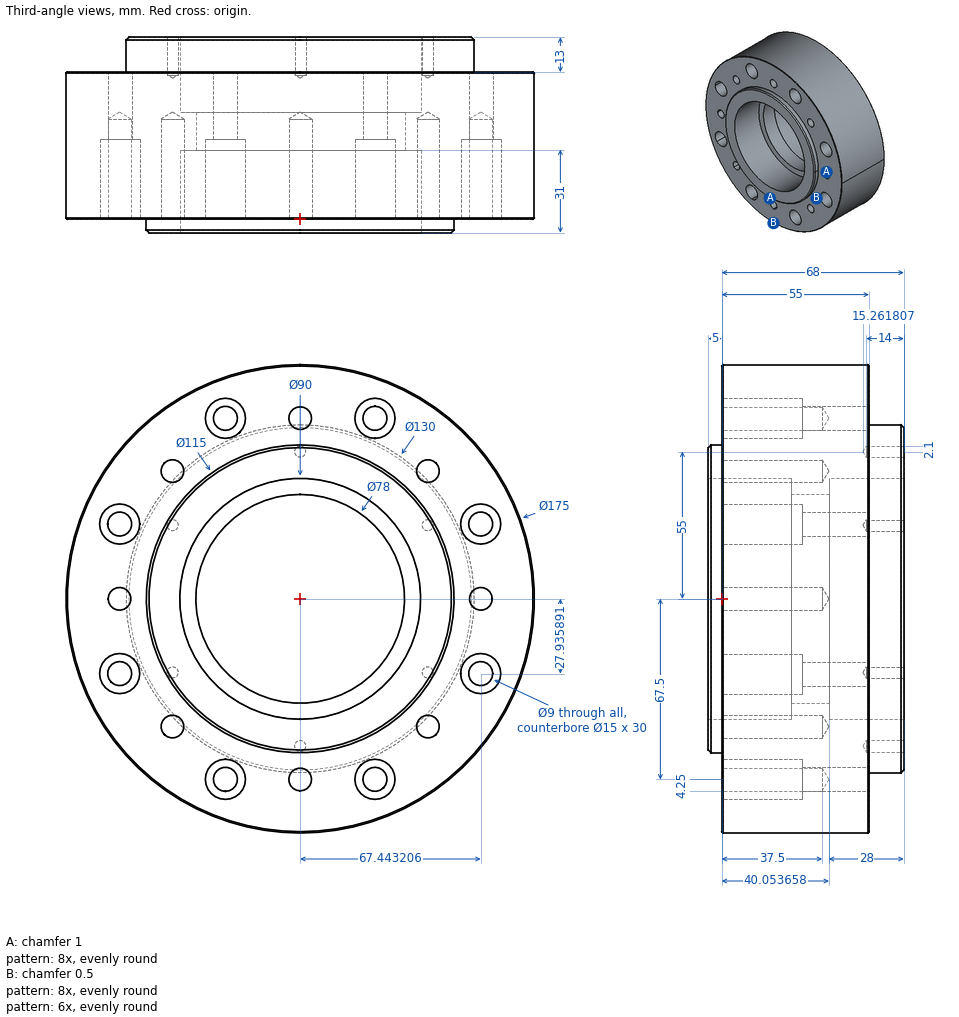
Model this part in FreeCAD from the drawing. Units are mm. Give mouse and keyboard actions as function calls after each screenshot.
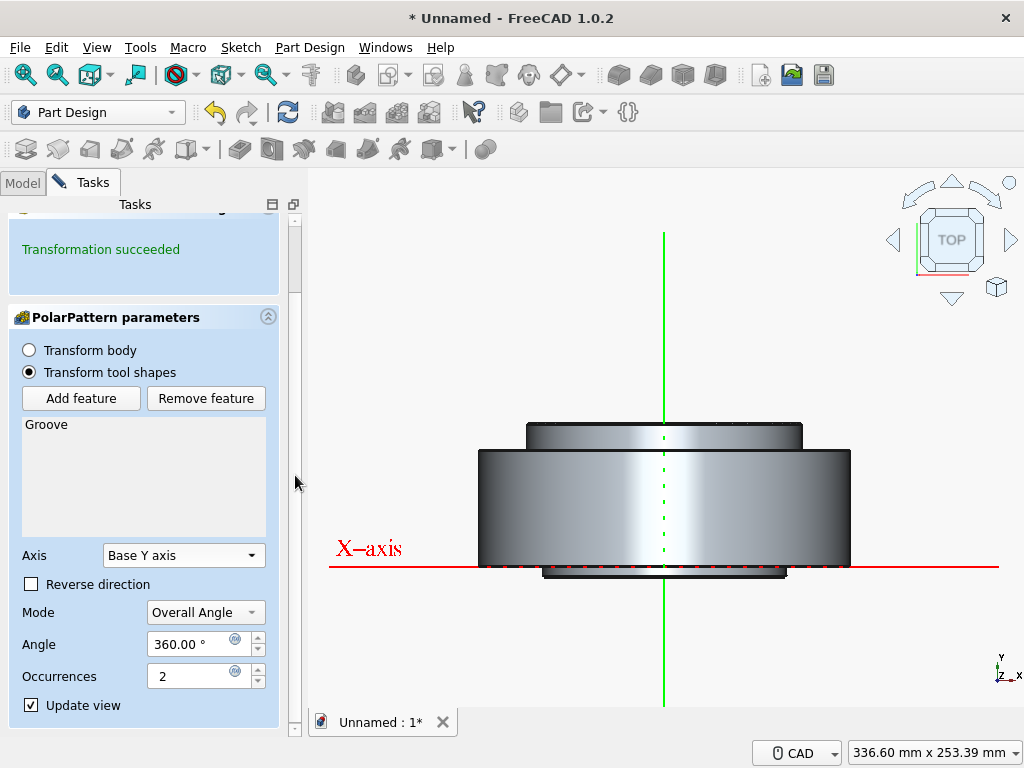
triple_click(198, 676)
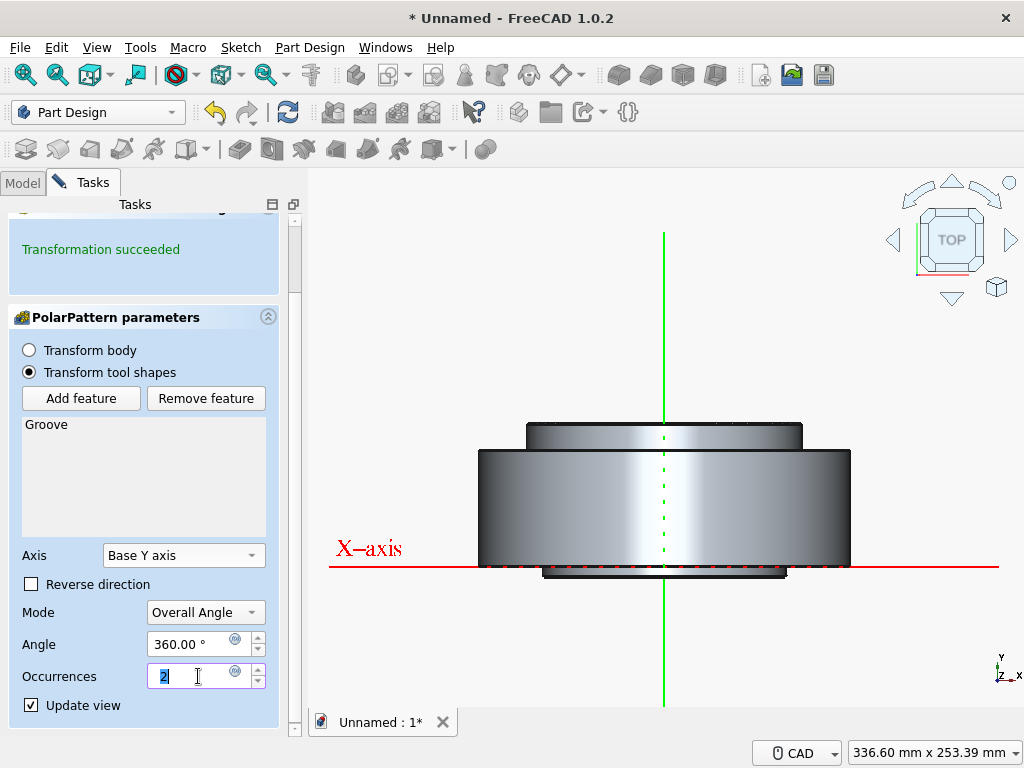
text(8)
key(Tab)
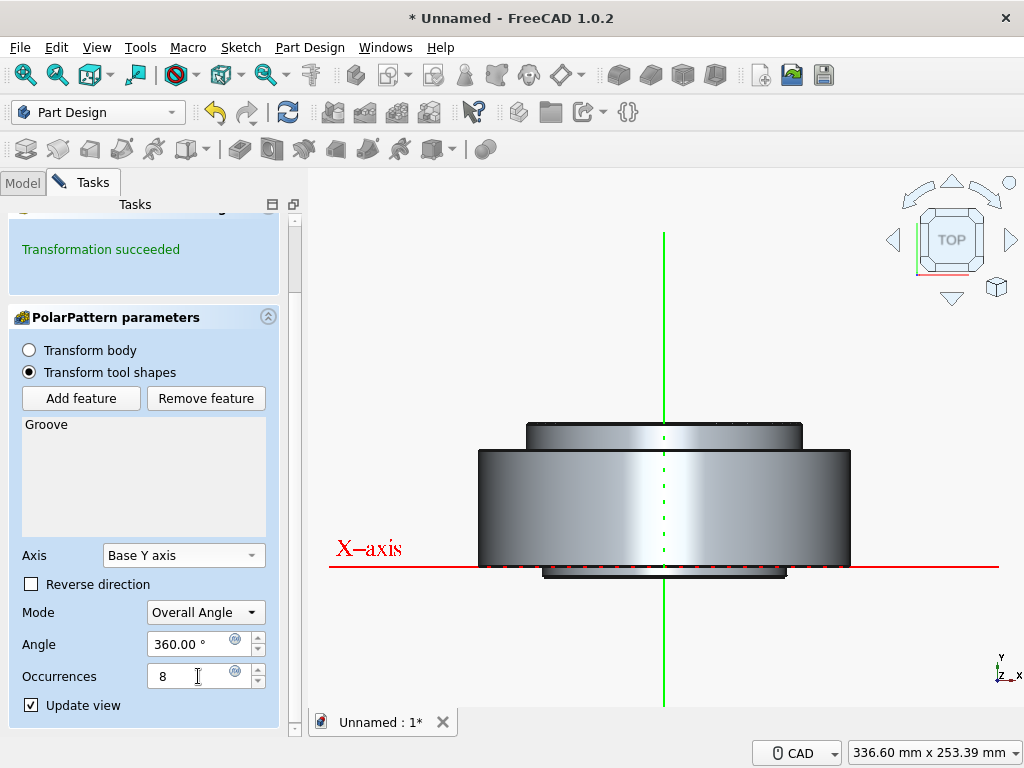
scroll(295, 475, up, 3)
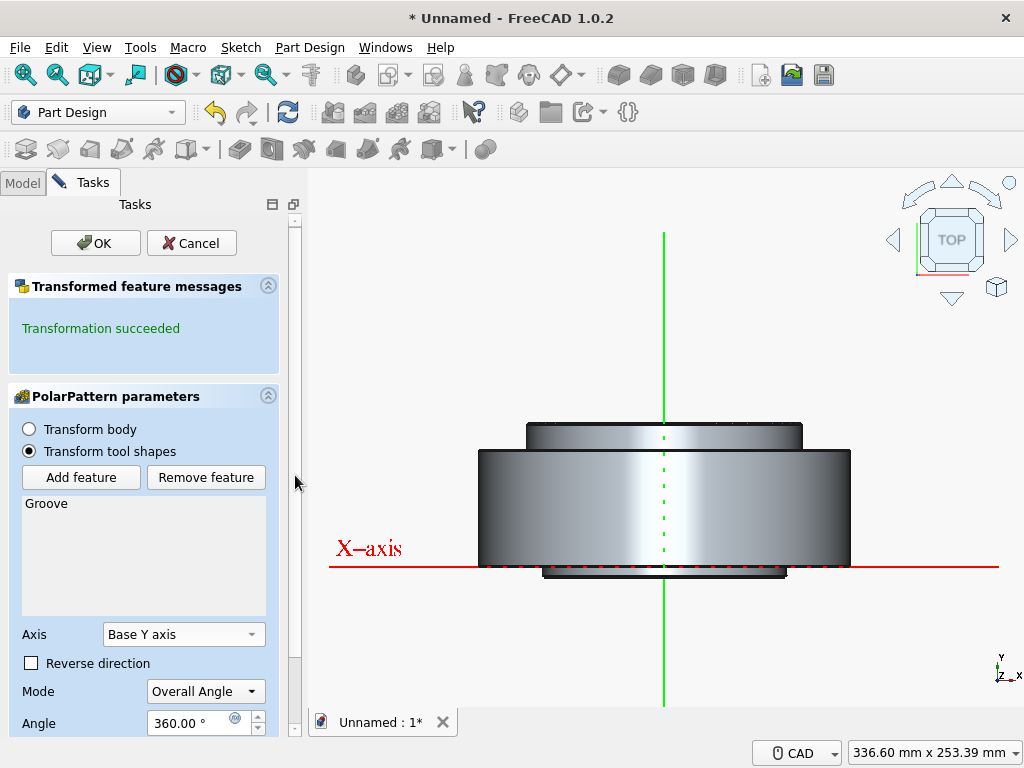
click(96, 243)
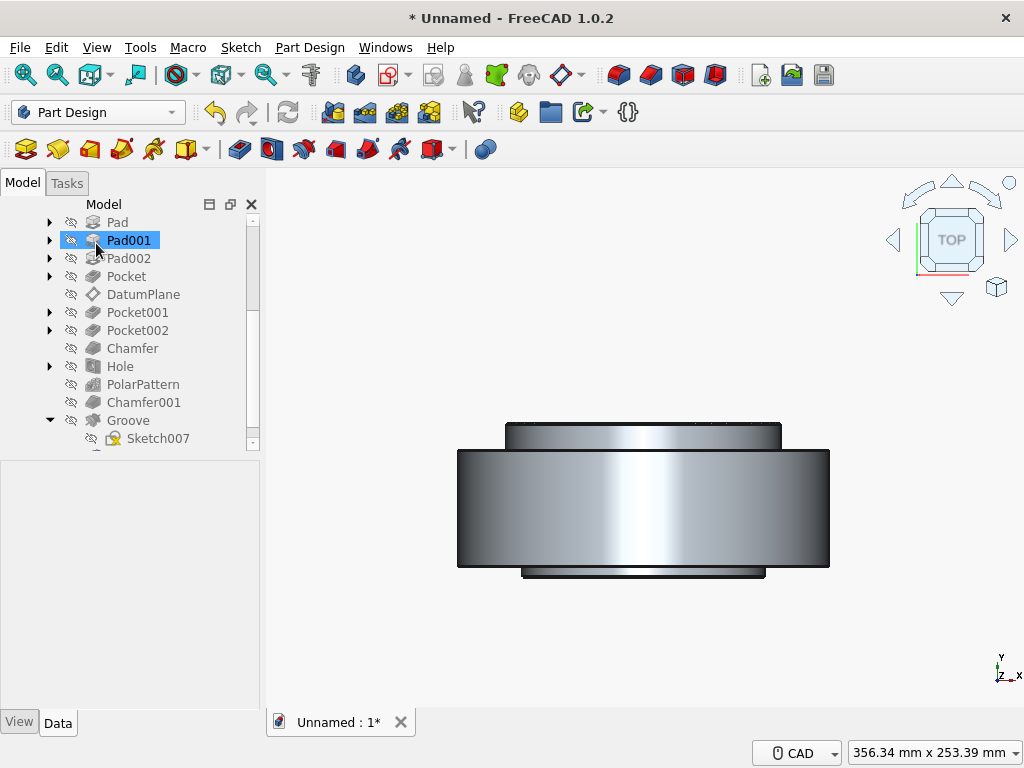
click(388, 76)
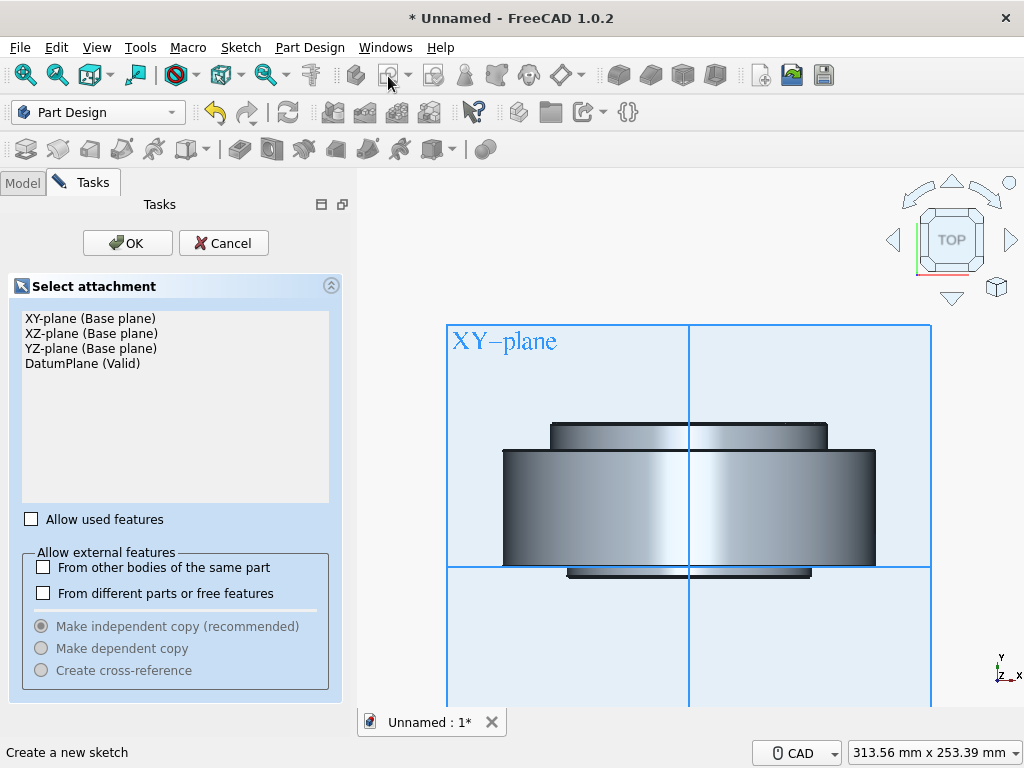
click(82, 348)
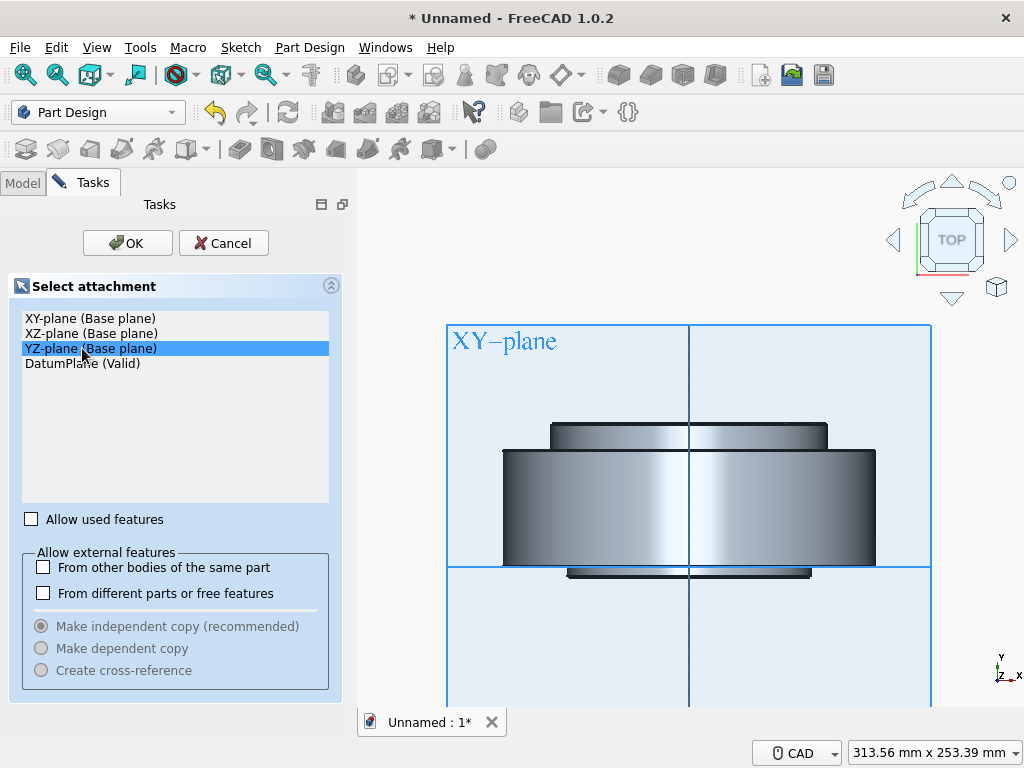
click(128, 243)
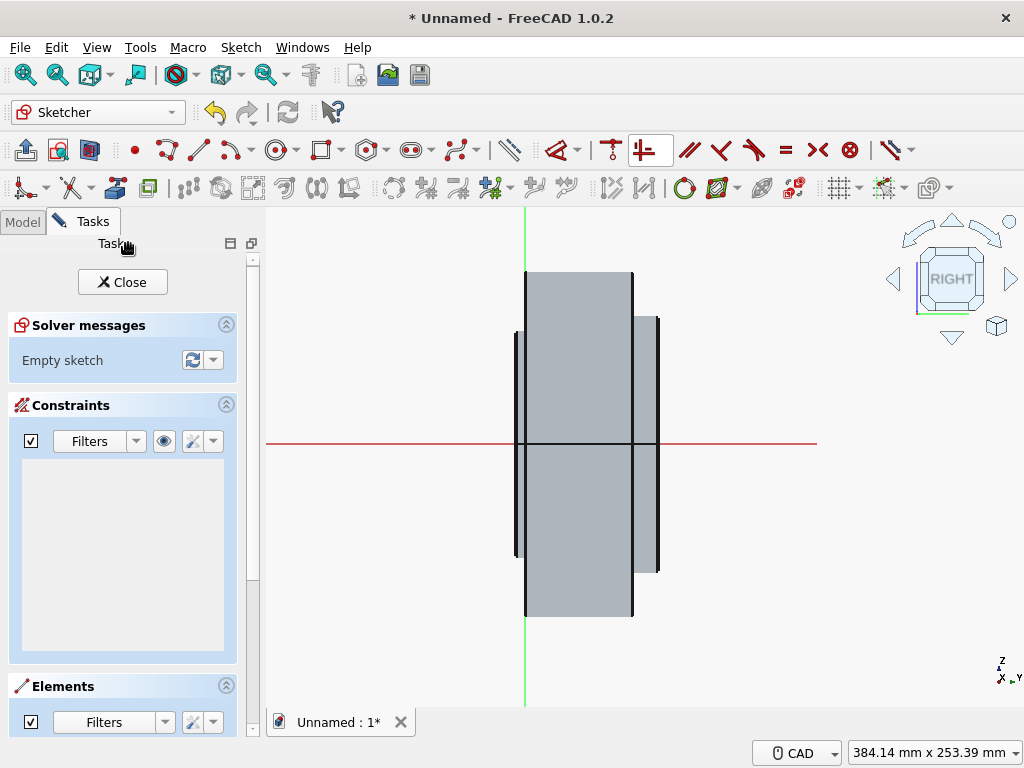
click(90, 150)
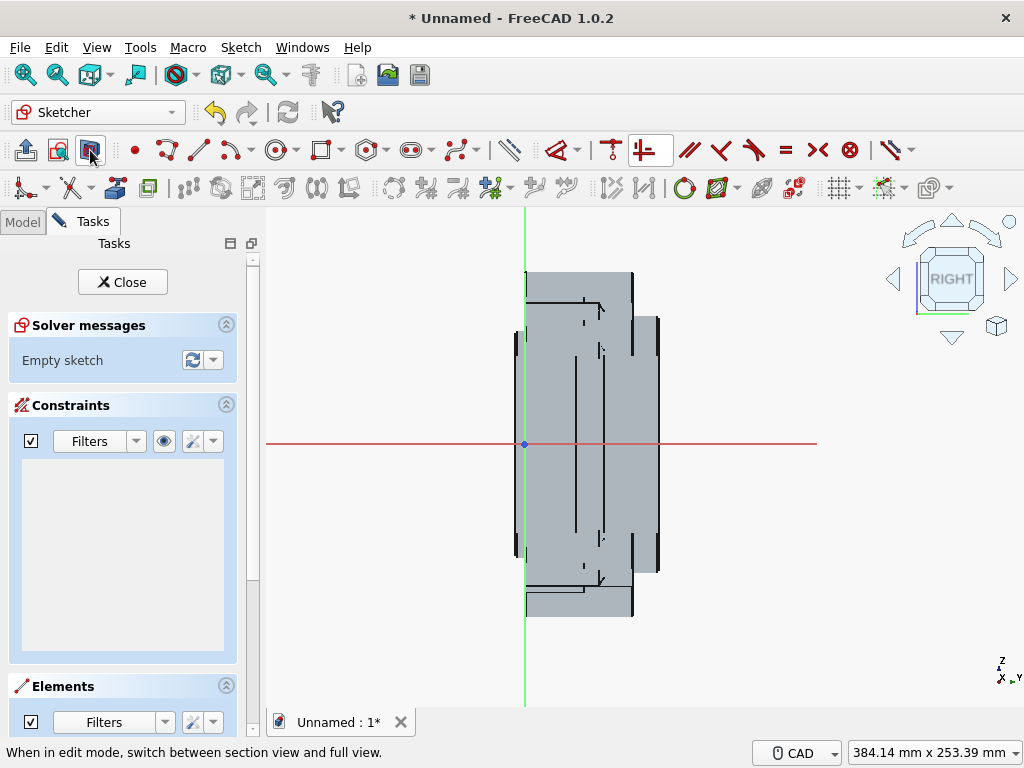
scroll(645, 319, up, 11)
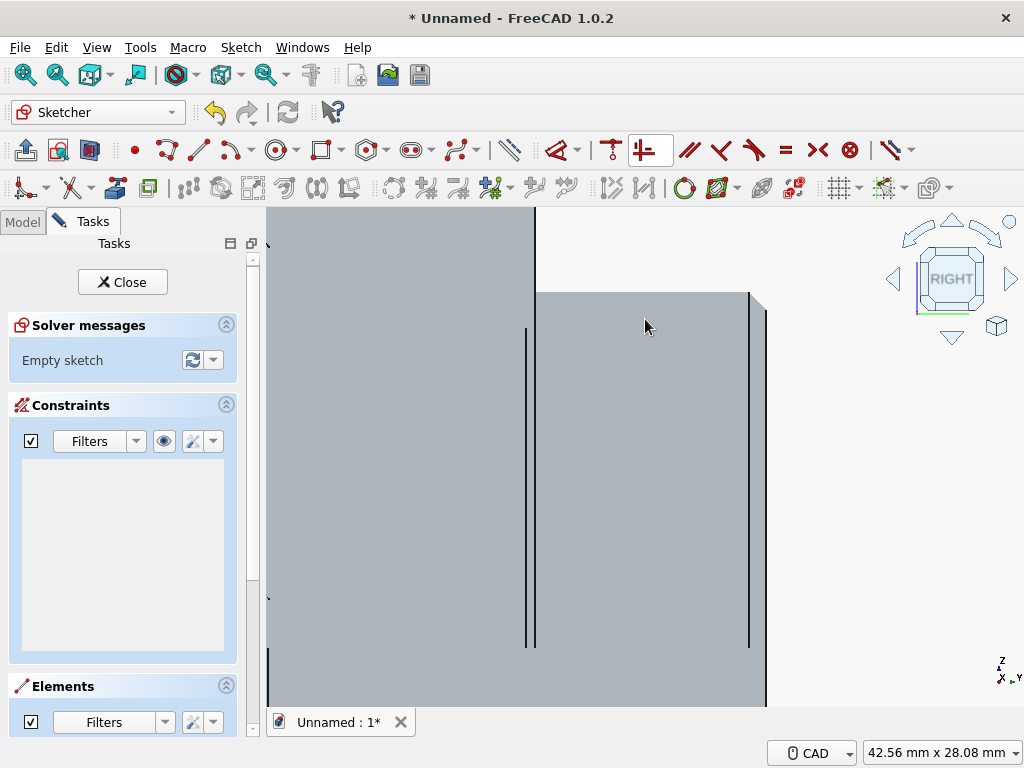
key(g)
key(m)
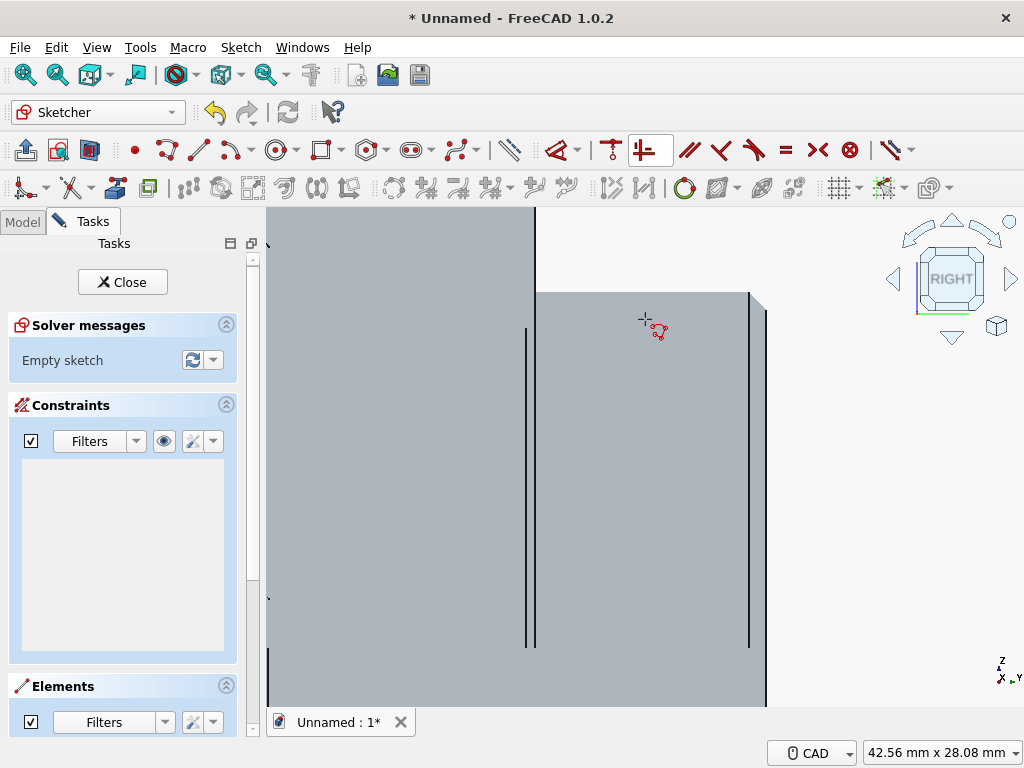
click(495, 470)
click(766, 470)
click(766, 433)
click(517, 433)
click(495, 471)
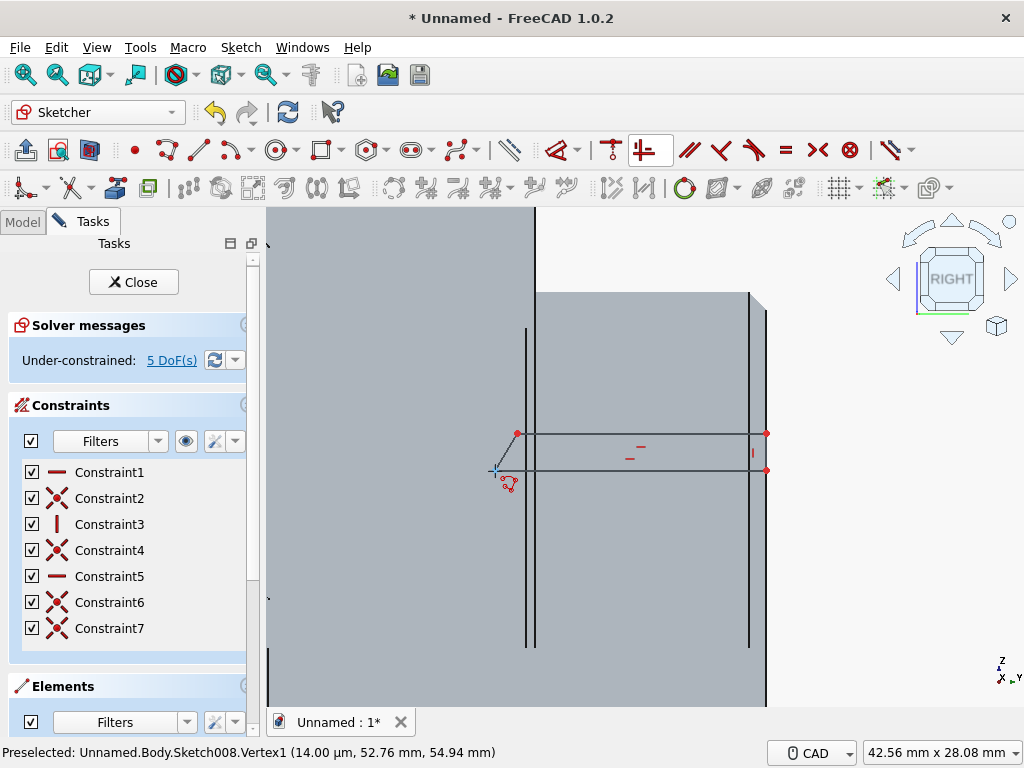
click(200, 150)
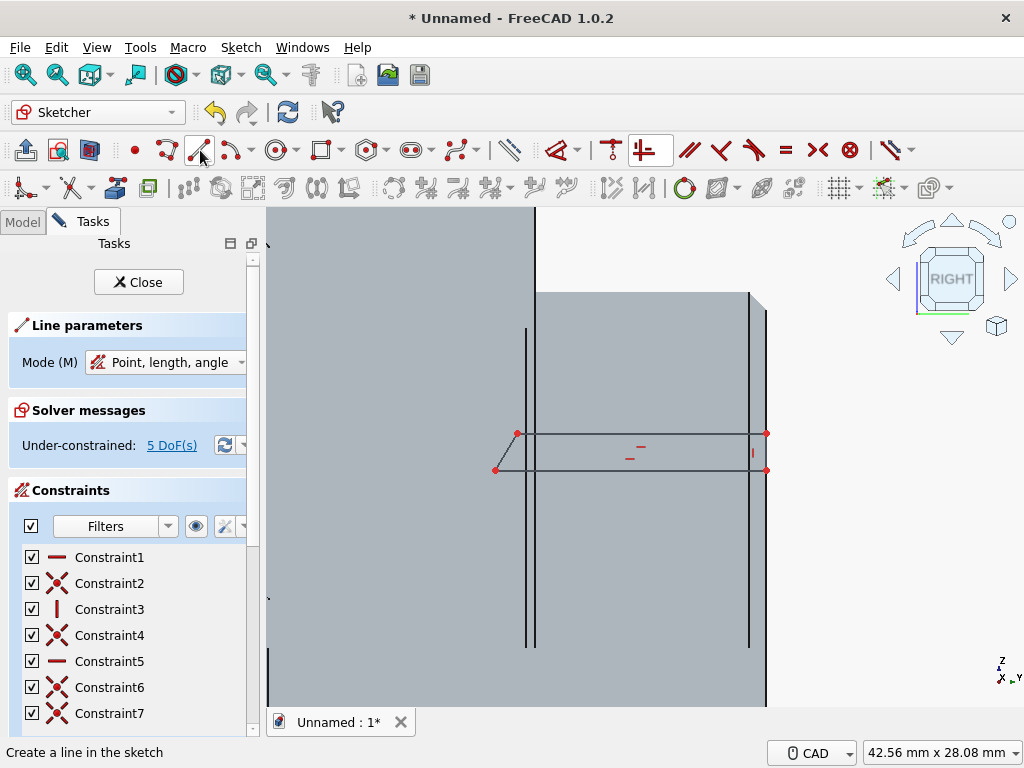
click(467, 470)
click(386, 470)
key(Escape)